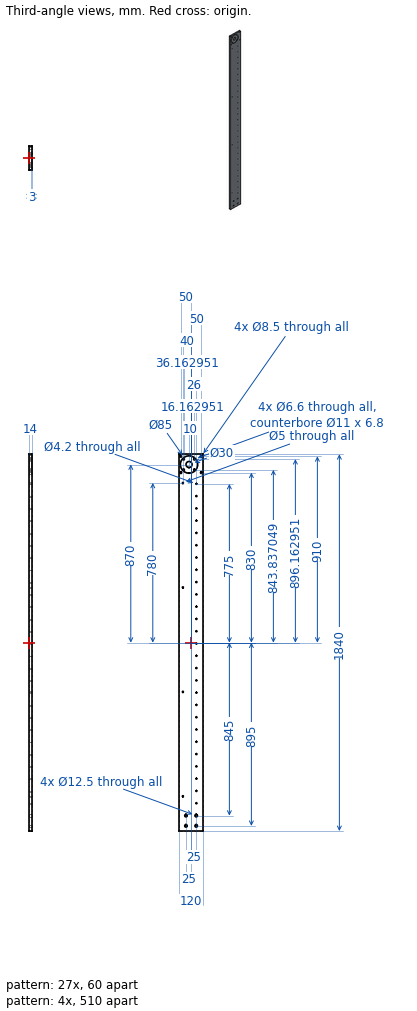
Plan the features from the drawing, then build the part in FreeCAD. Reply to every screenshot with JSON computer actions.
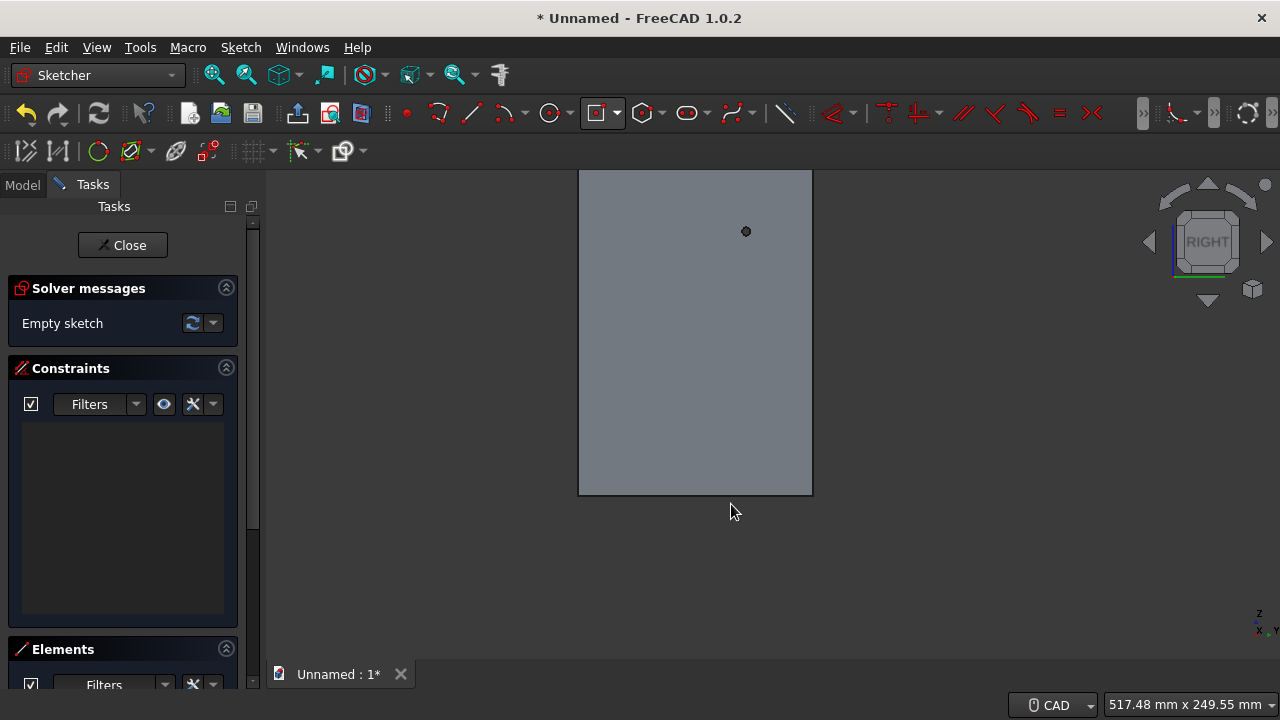
{"action": "scroll", "coordinate": [690, 388], "scroll_direction": "up", "scroll_amount": 5}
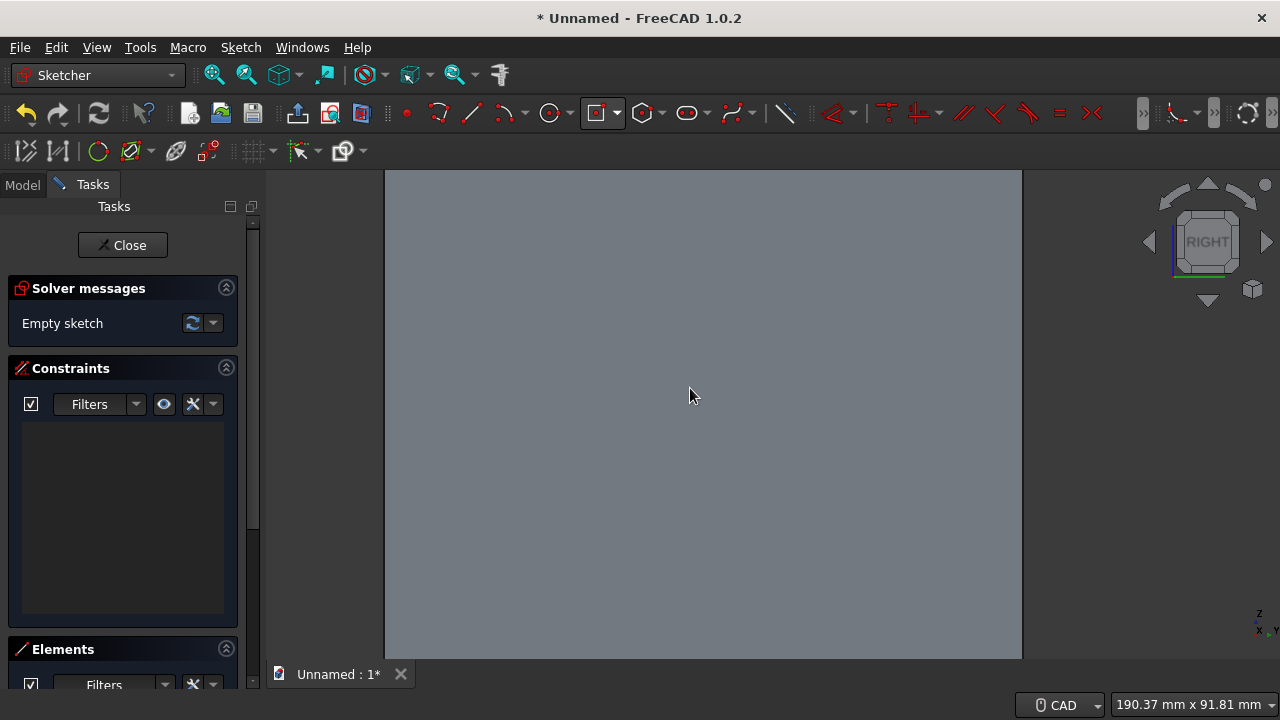
{"action": "left_click", "coordinate": [550, 114]}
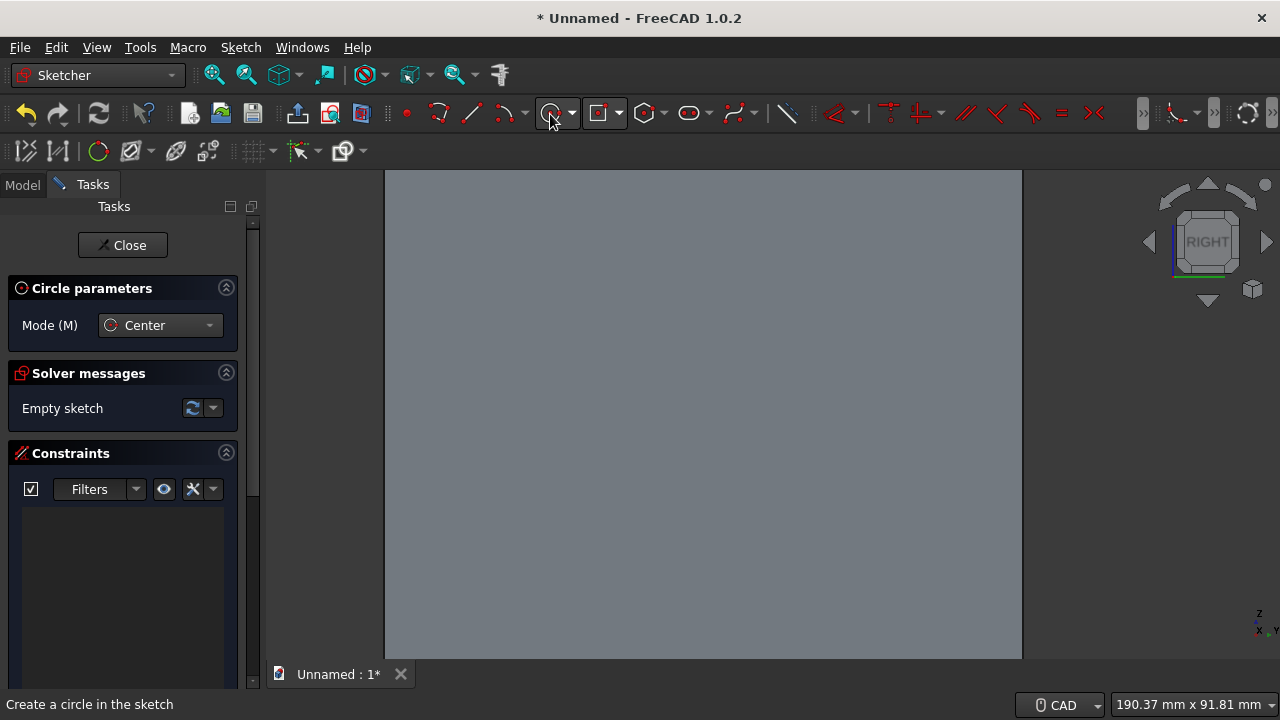
{"action": "left_click", "coordinate": [837, 281]}
{"action": "mouse_move", "coordinate": [860, 258]}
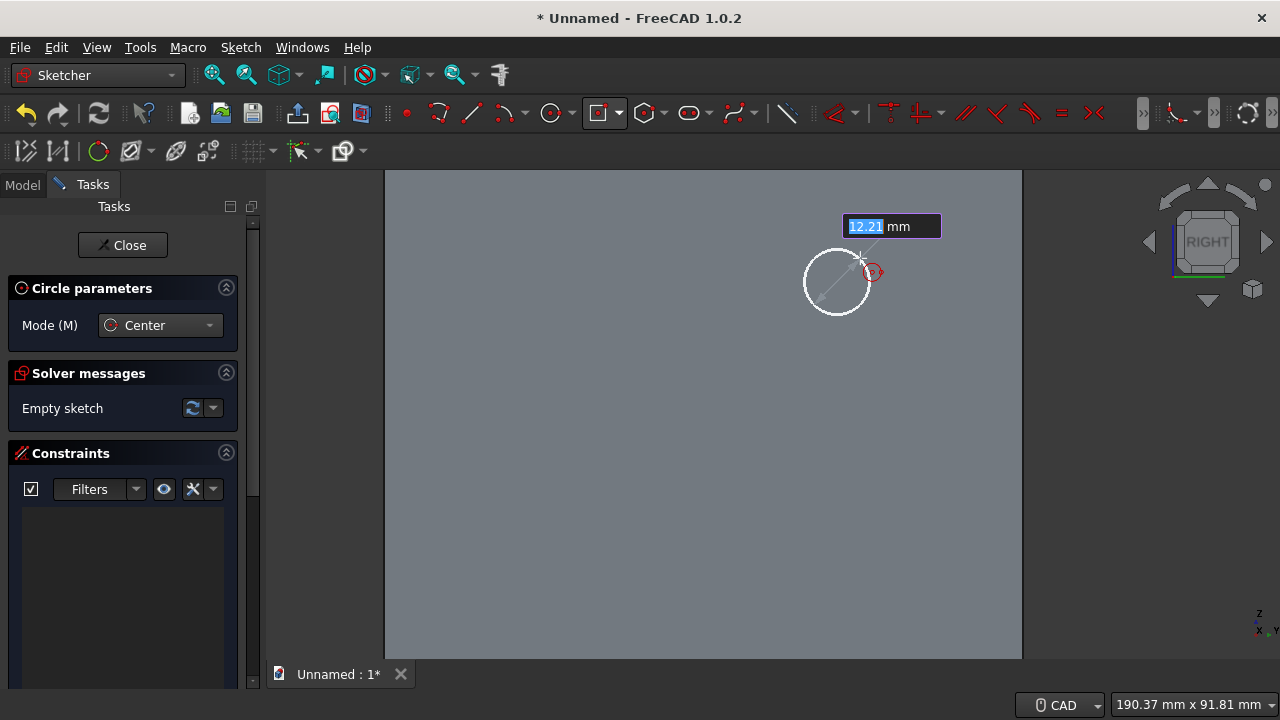
{"action": "type", "text": "12.5"}
{"action": "key", "text": "Return"}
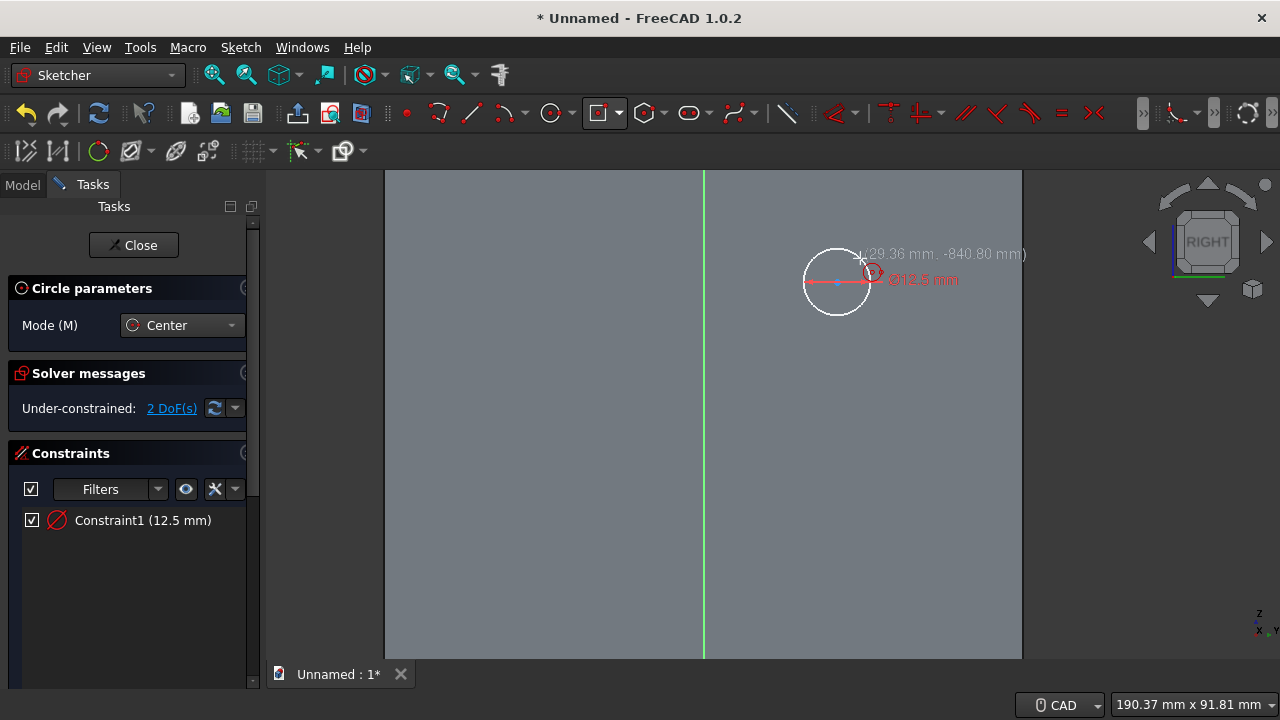
{"action": "left_click", "coordinate": [837, 548]}
{"action": "mouse_move", "coordinate": [860, 524]}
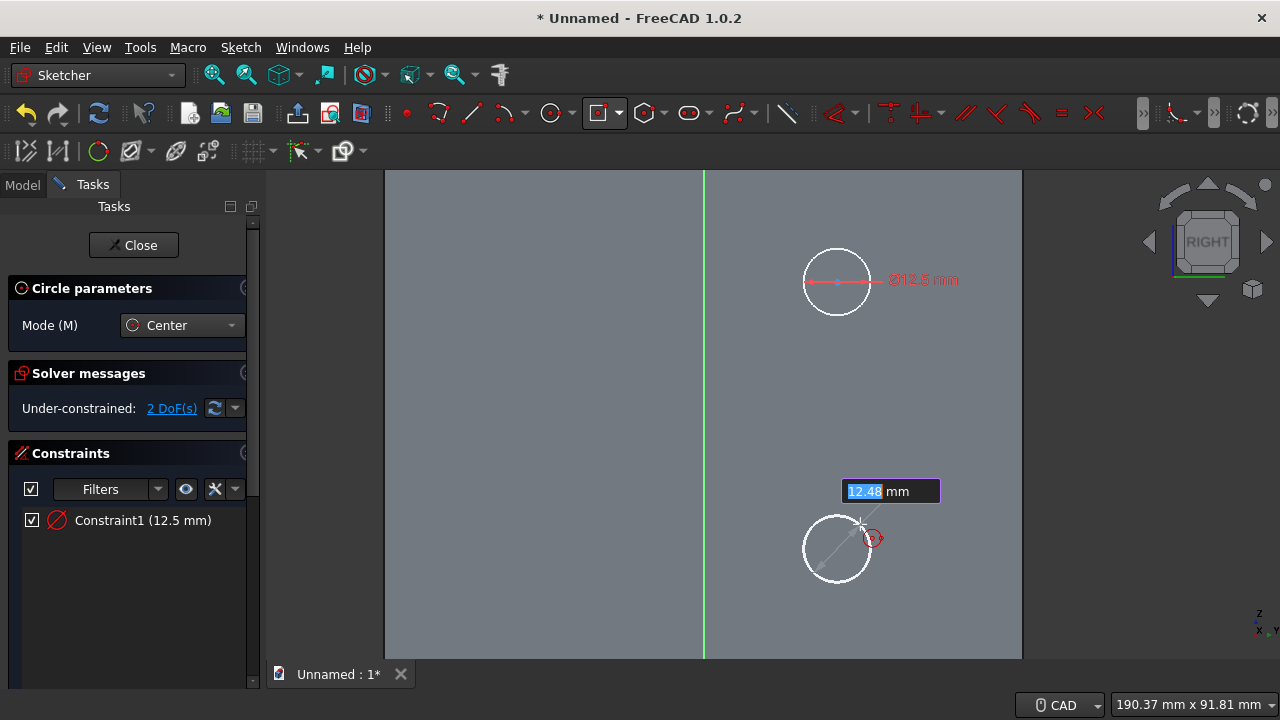
{"action": "type", "text": "12.5"}
{"action": "key", "text": "Return"}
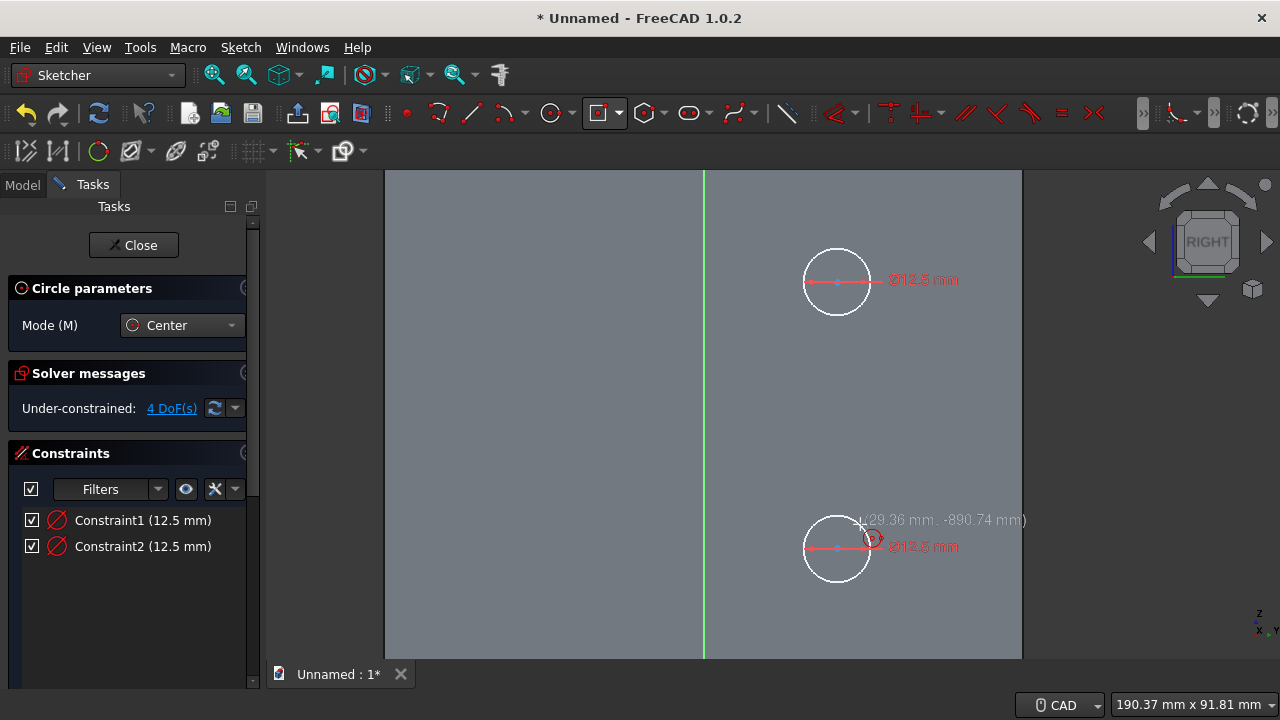
{"action": "left_click", "coordinate": [570, 281]}
{"action": "mouse_move", "coordinate": [594, 258]}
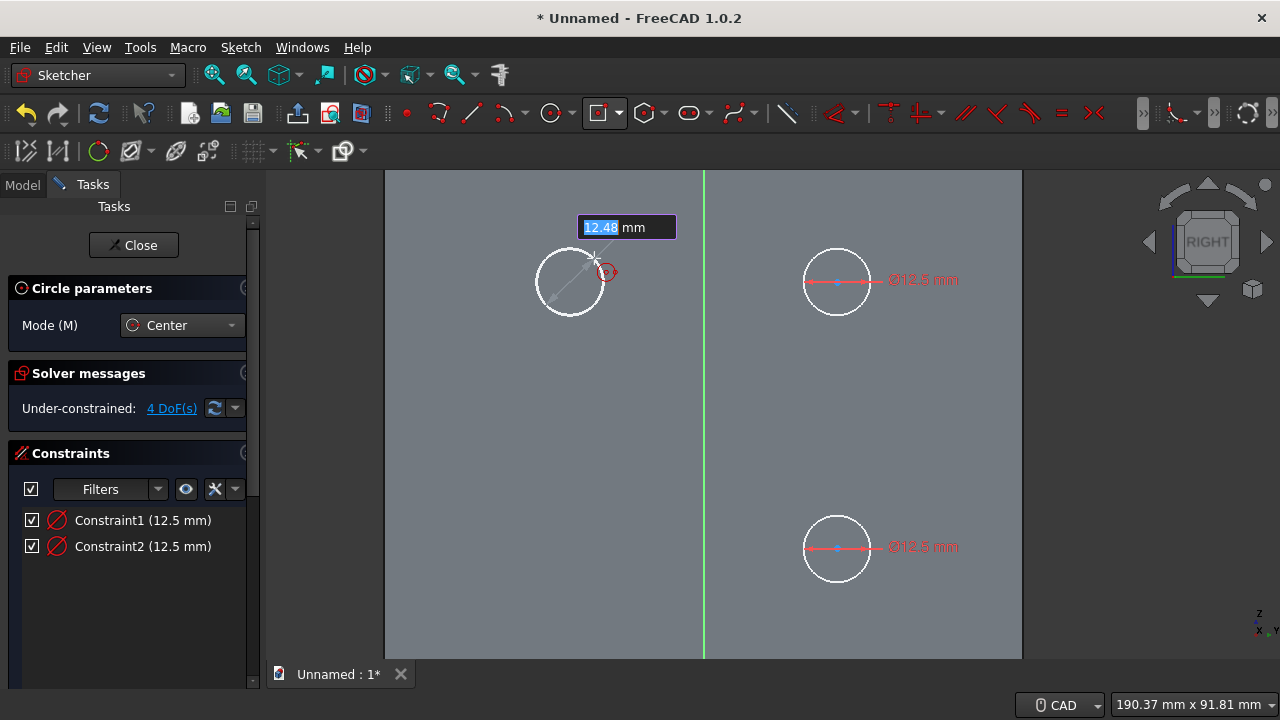
{"action": "type", "text": "12.5"}
{"action": "key", "text": "Return"}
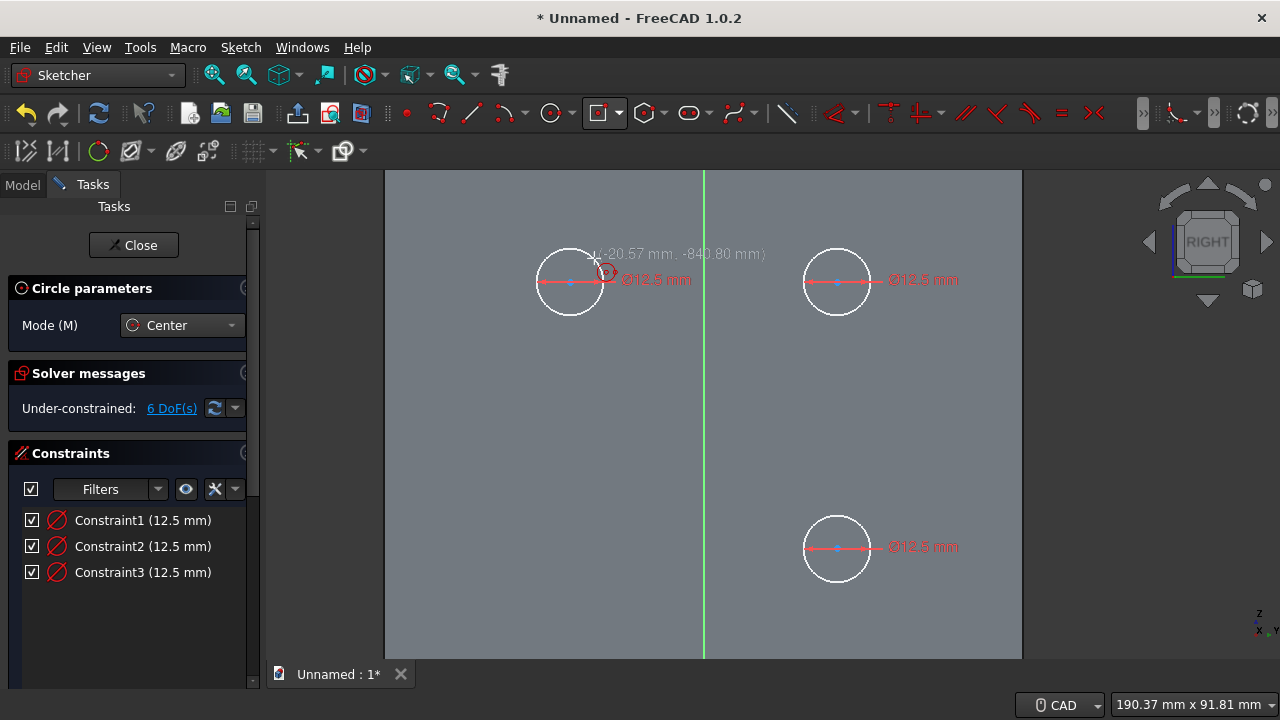
{"action": "left_click", "coordinate": [570, 548]}
{"action": "mouse_move", "coordinate": [594, 524]}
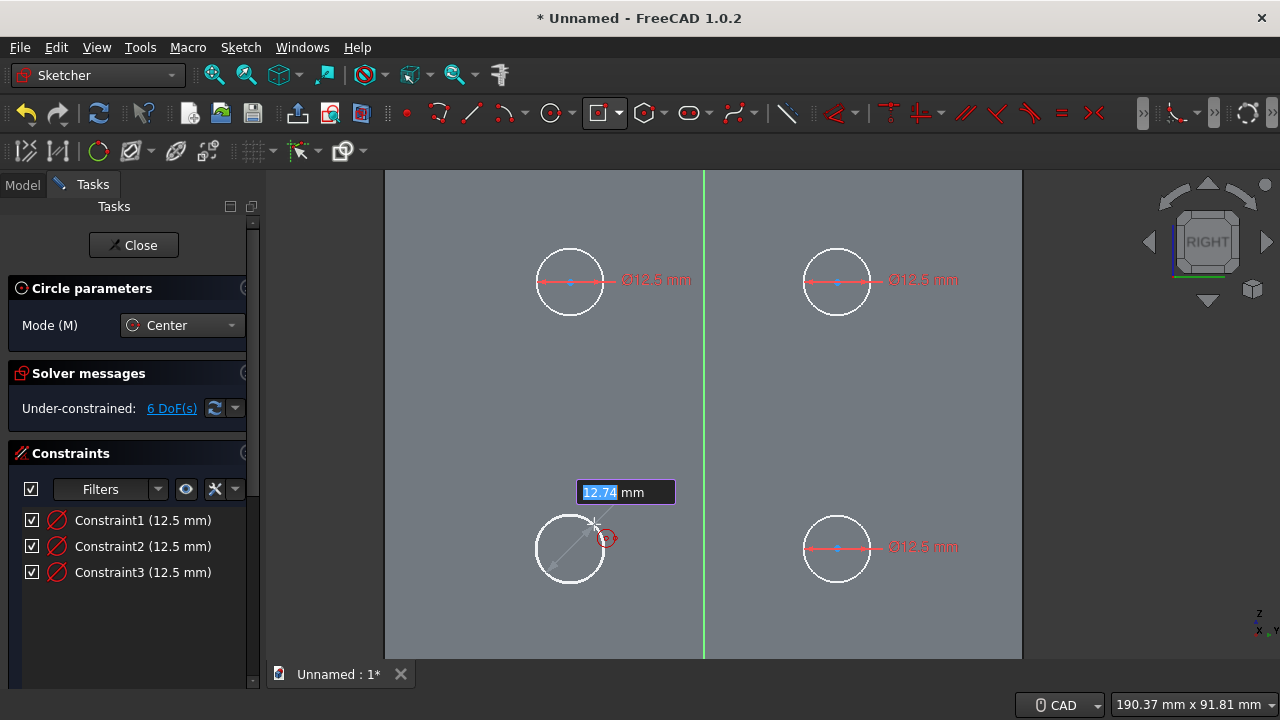
{"action": "type", "text": "12.5"}
{"action": "key", "text": "Return"}
{"action": "key", "text": "Escape"}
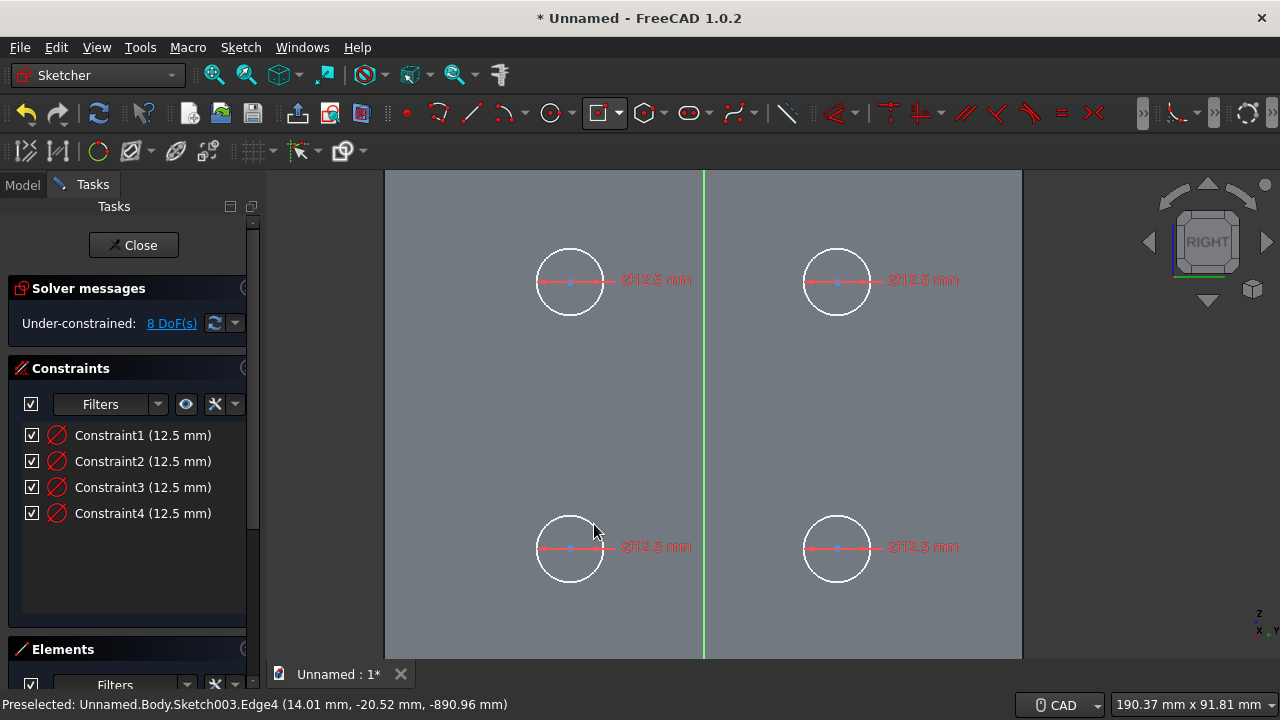
{"action": "left_click", "coordinate": [837, 282]}